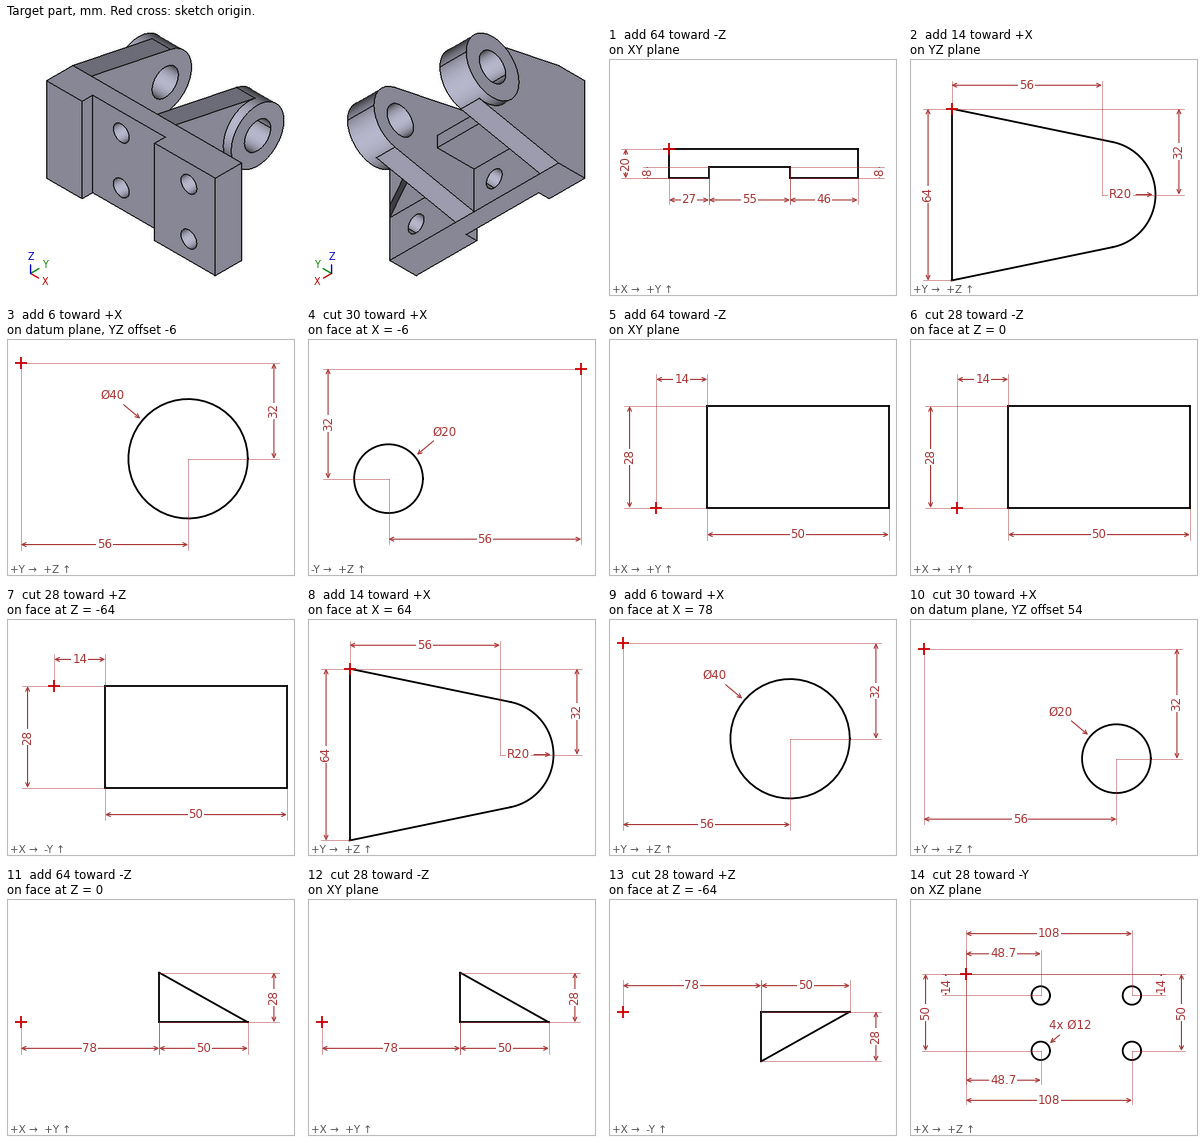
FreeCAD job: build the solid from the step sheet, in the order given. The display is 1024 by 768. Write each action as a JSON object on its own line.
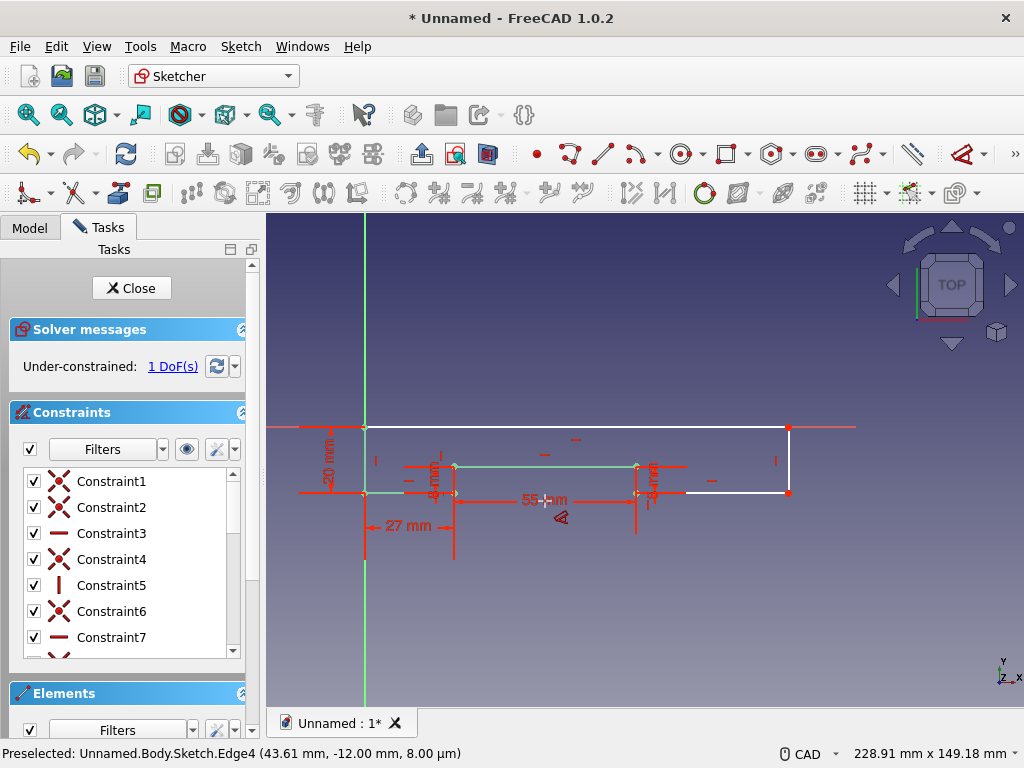
{"action": "left_click", "coordinate": [682, 493]}
{"action": "left_click", "coordinate": [713, 527]}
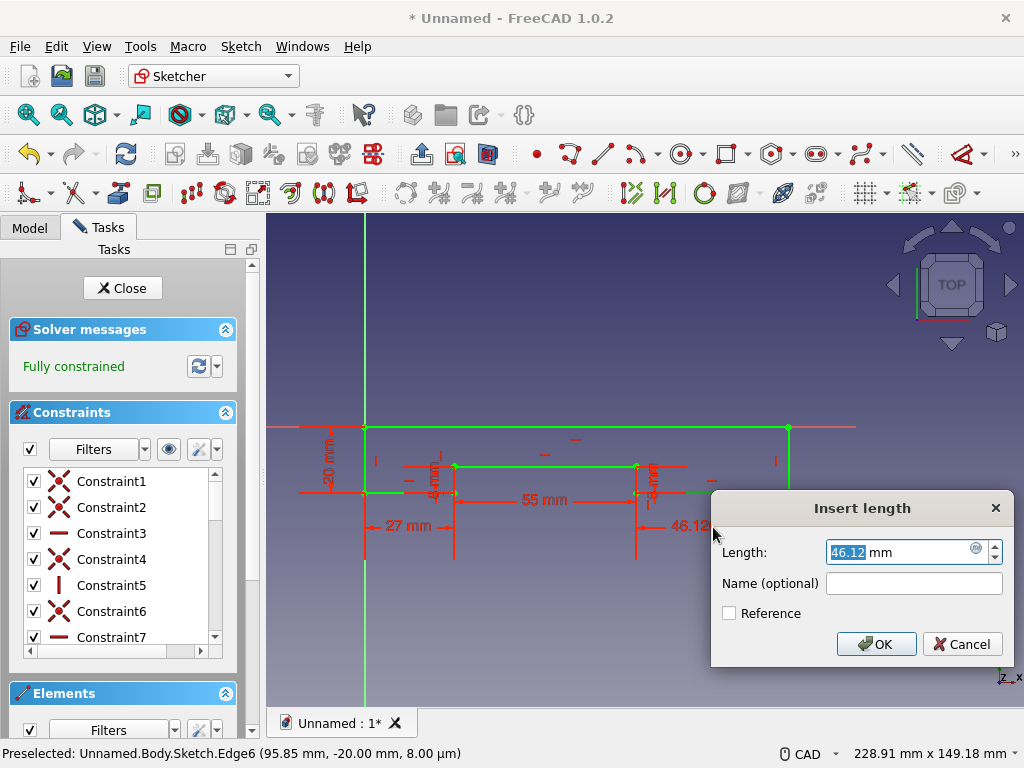
{"action": "type", "text": "46"}
{"action": "key", "text": "Return"}
{"action": "key", "text": "Escape"}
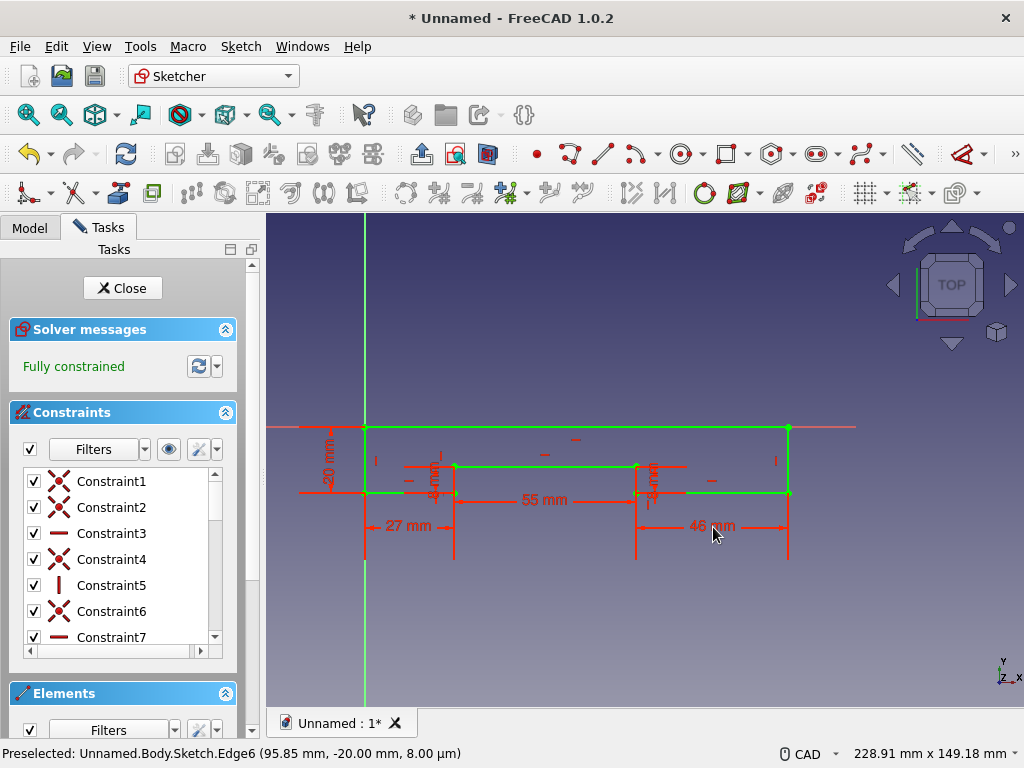
{"action": "left_click", "coordinate": [123, 288]}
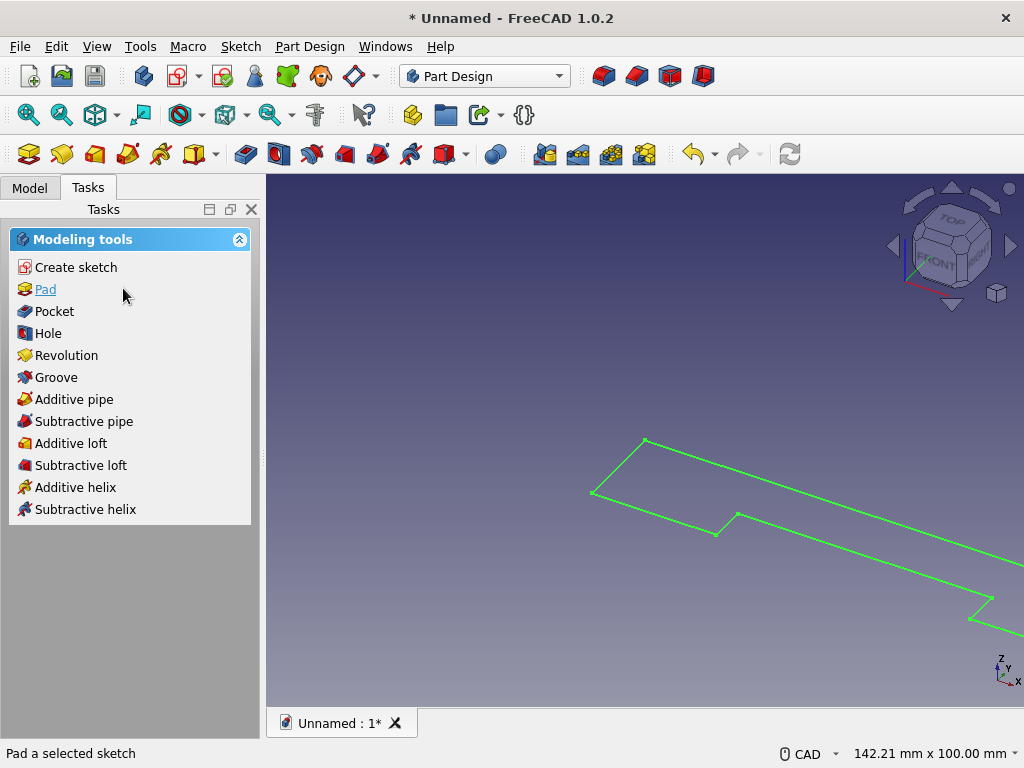
{"action": "left_click", "coordinate": [29, 154]}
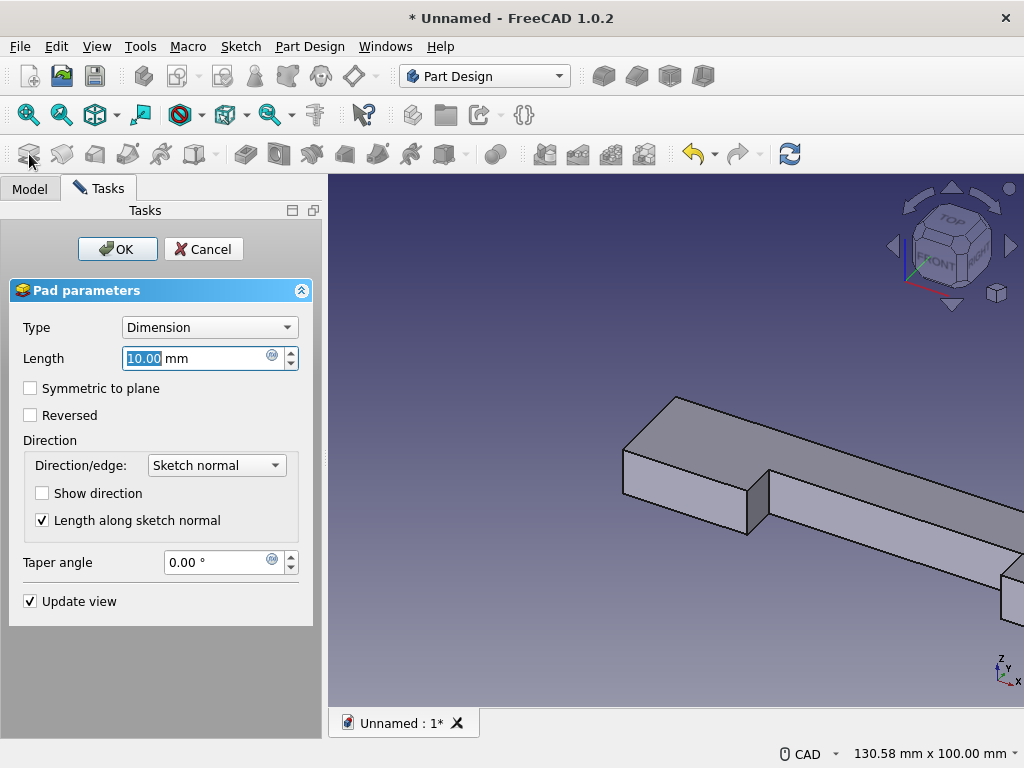
{"action": "type", "text": "64"}
{"action": "key", "text": "Tab"}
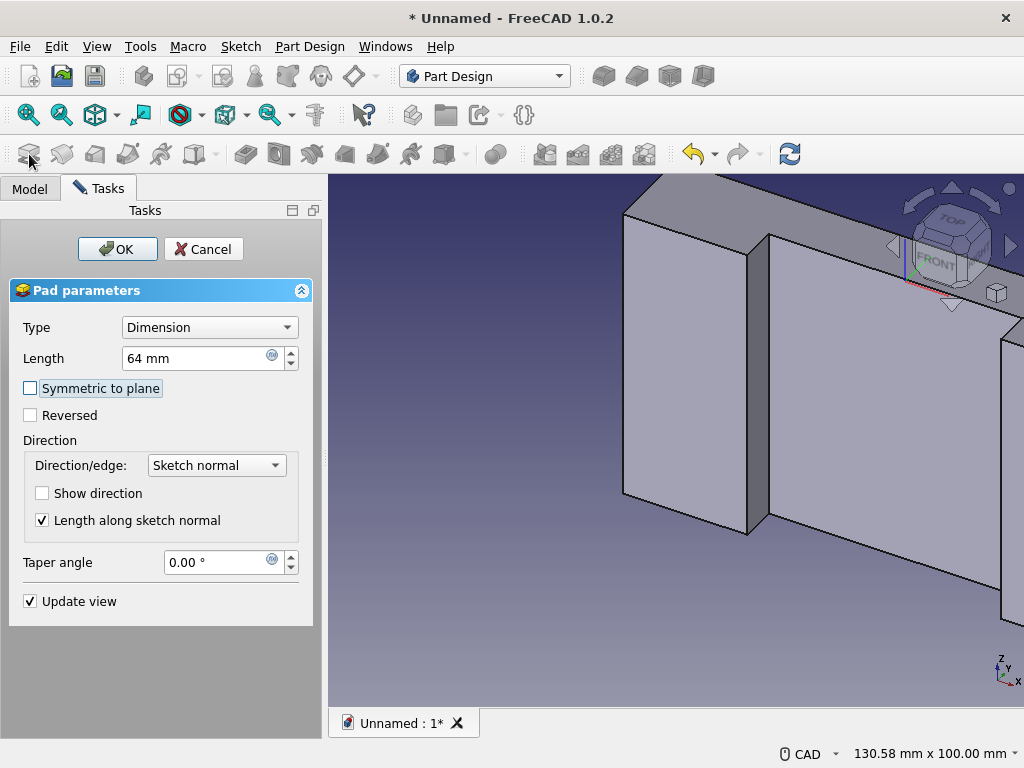
{"action": "left_click", "coordinate": [31, 415]}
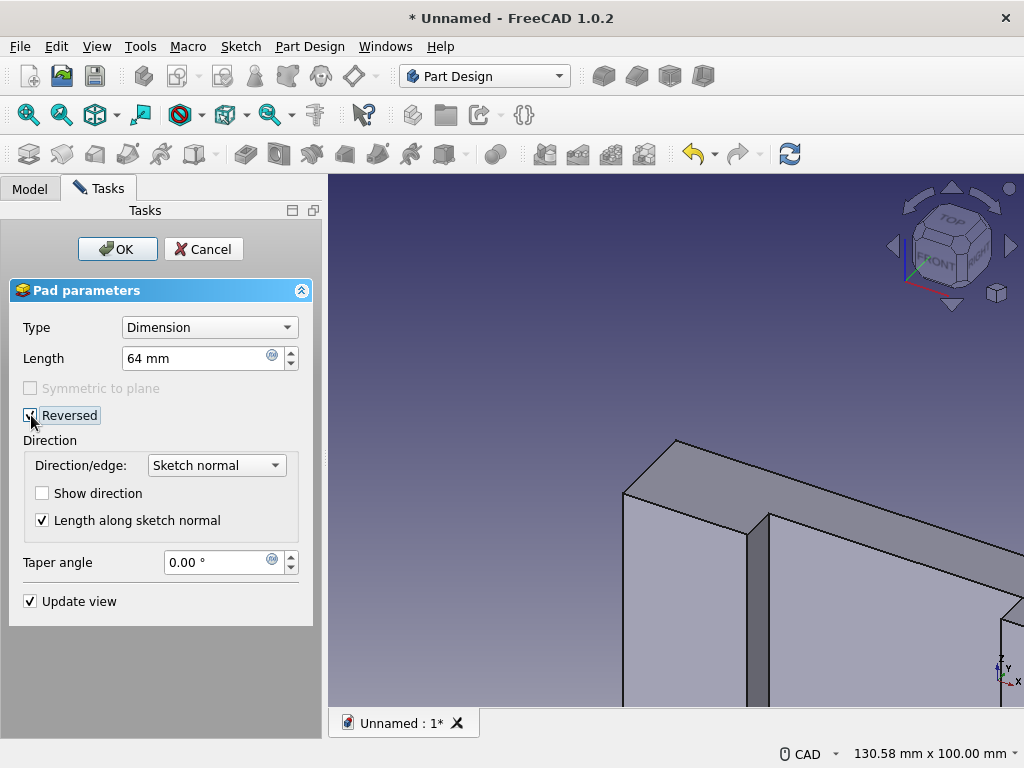
{"action": "left_click", "coordinate": [118, 249]}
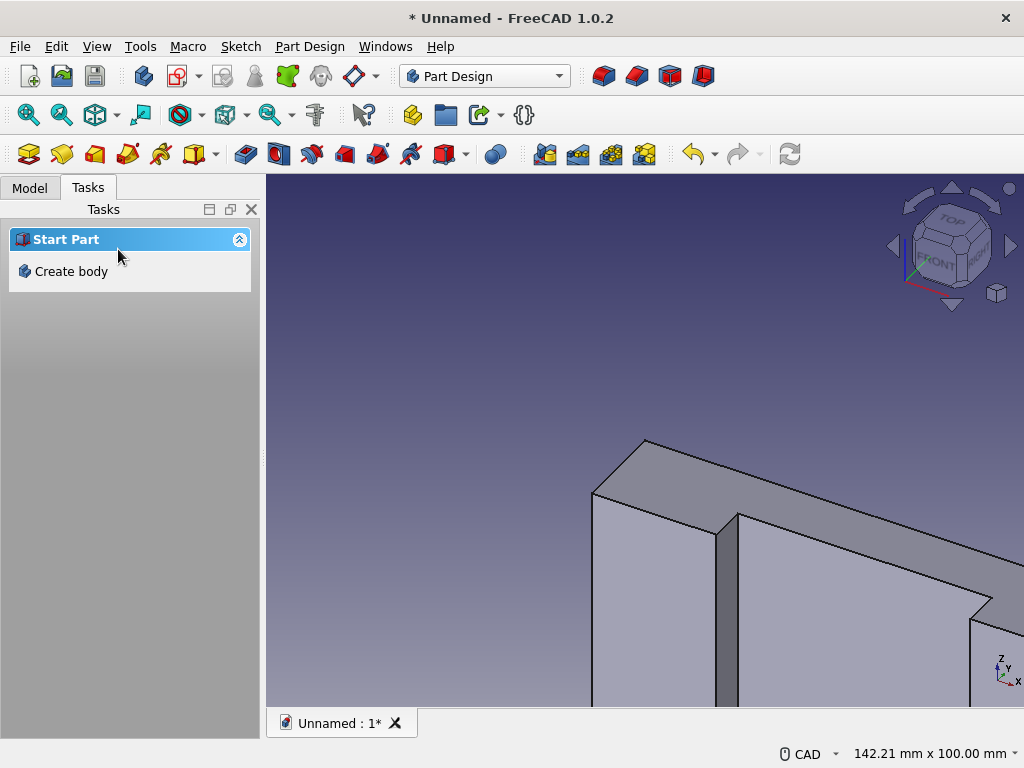
{"action": "left_click", "coordinate": [29, 116]}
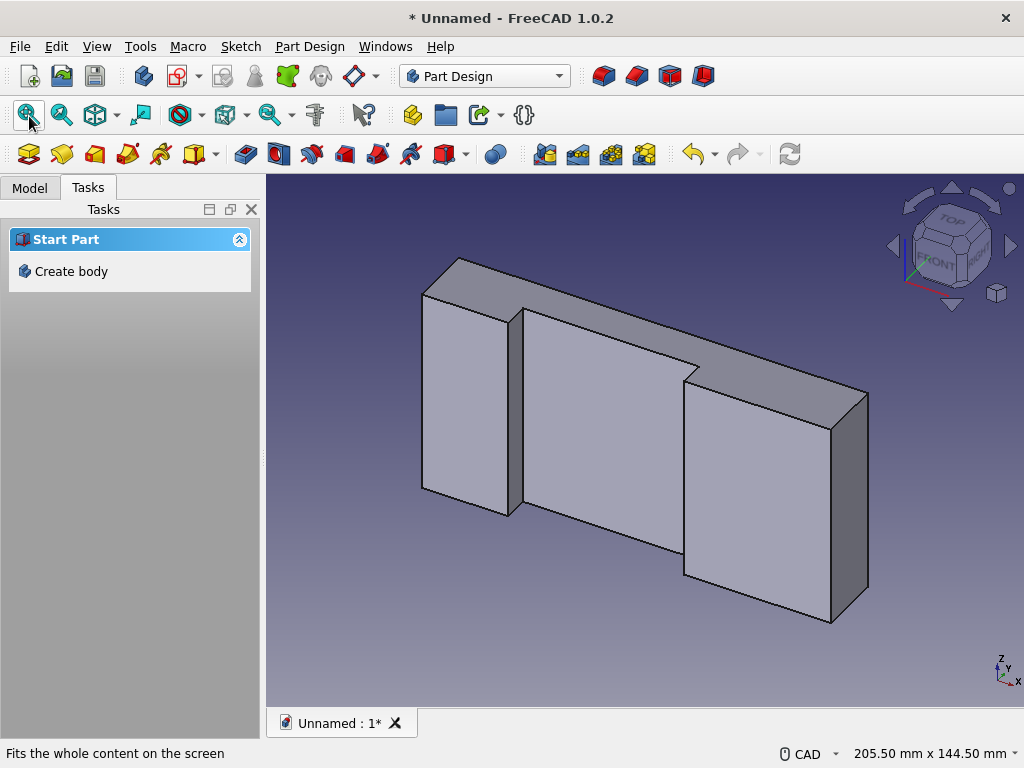
{"action": "left_click", "coordinate": [176, 76]}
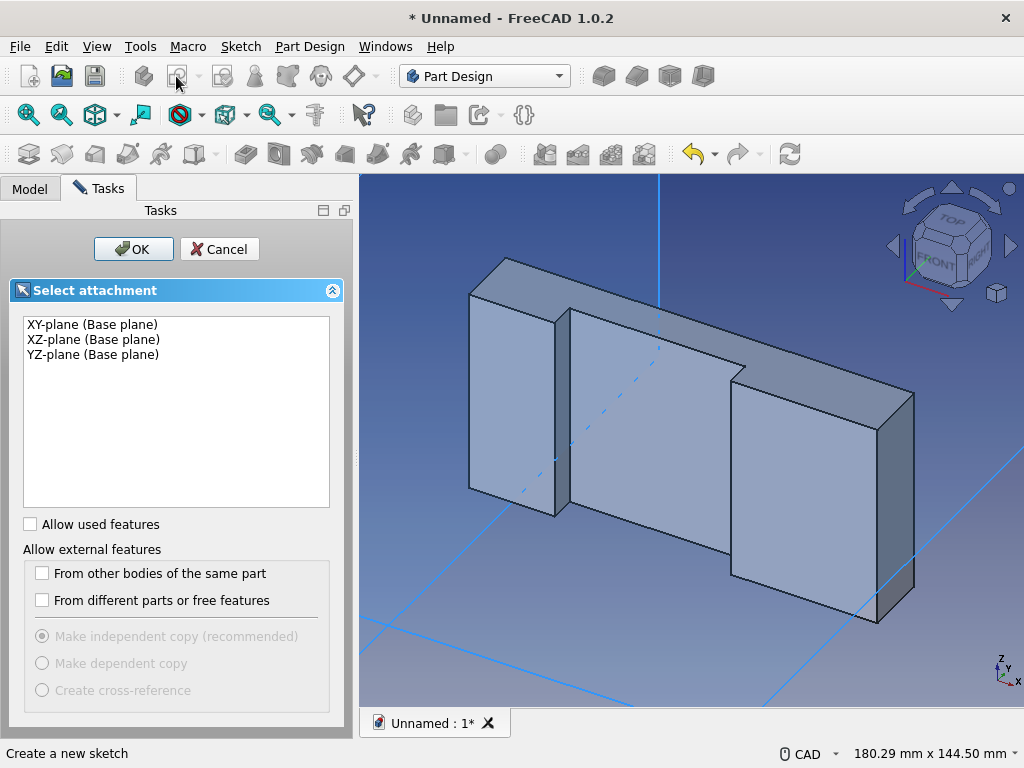
{"action": "left_click", "coordinate": [84, 354]}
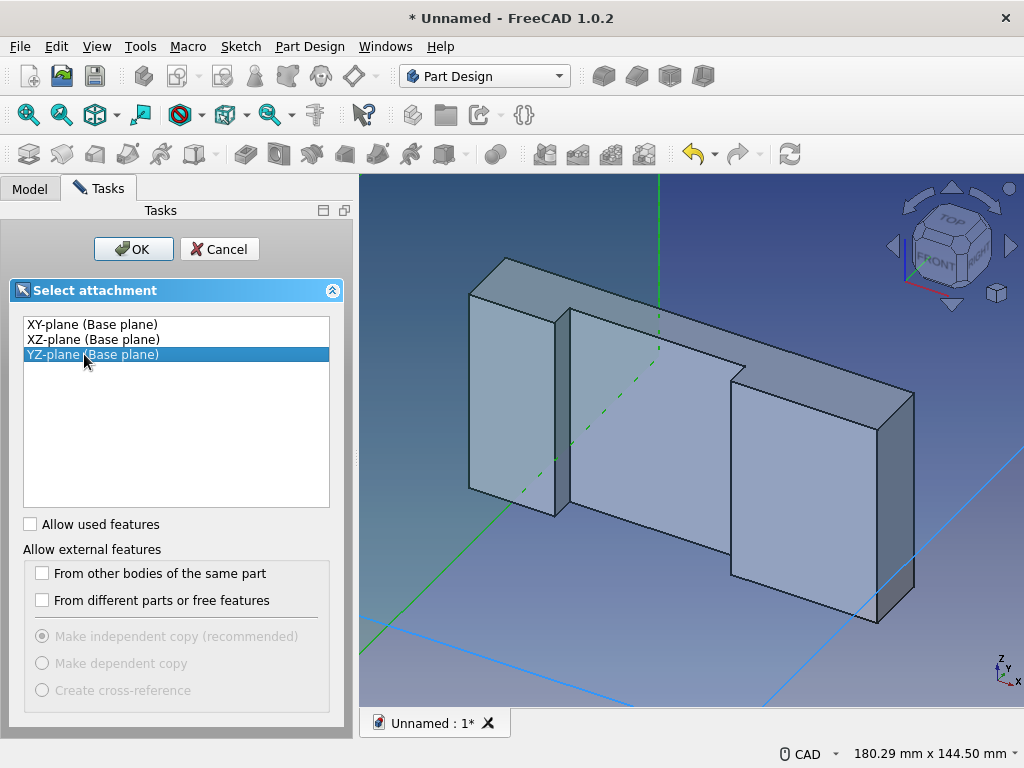
{"action": "left_click", "coordinate": [134, 249]}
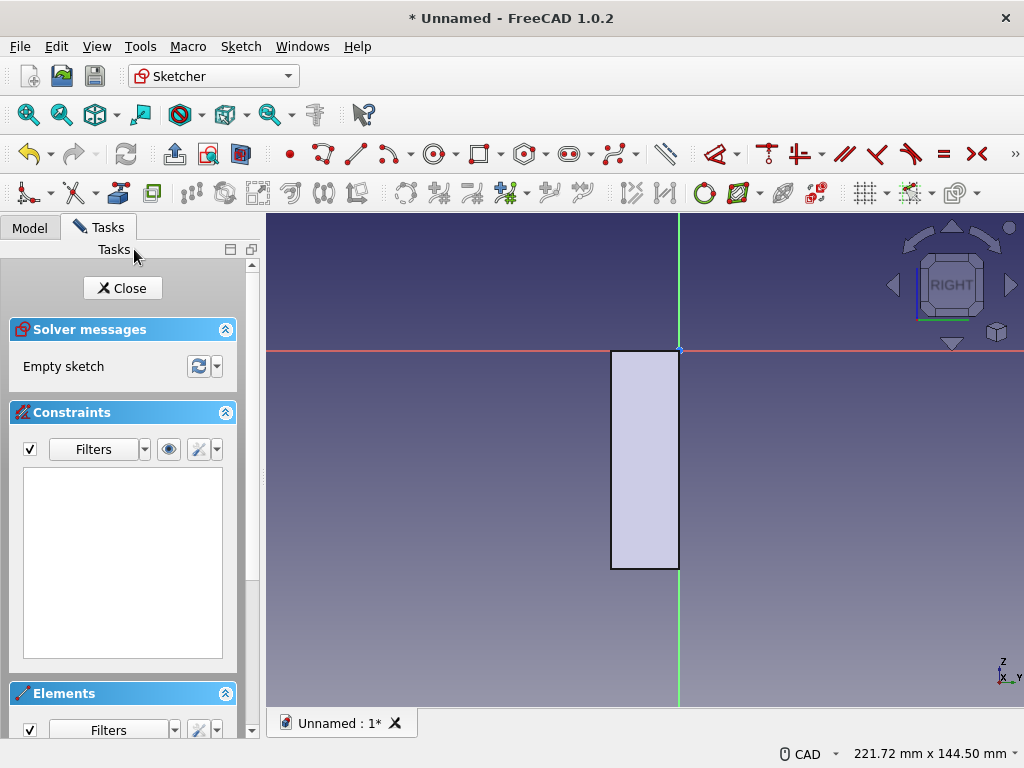
{"action": "left_click", "coordinate": [241, 154]}